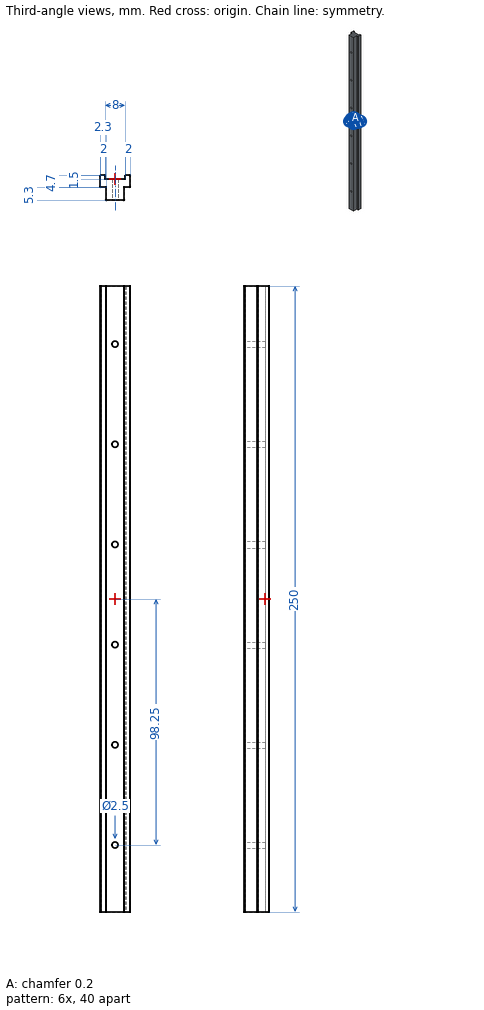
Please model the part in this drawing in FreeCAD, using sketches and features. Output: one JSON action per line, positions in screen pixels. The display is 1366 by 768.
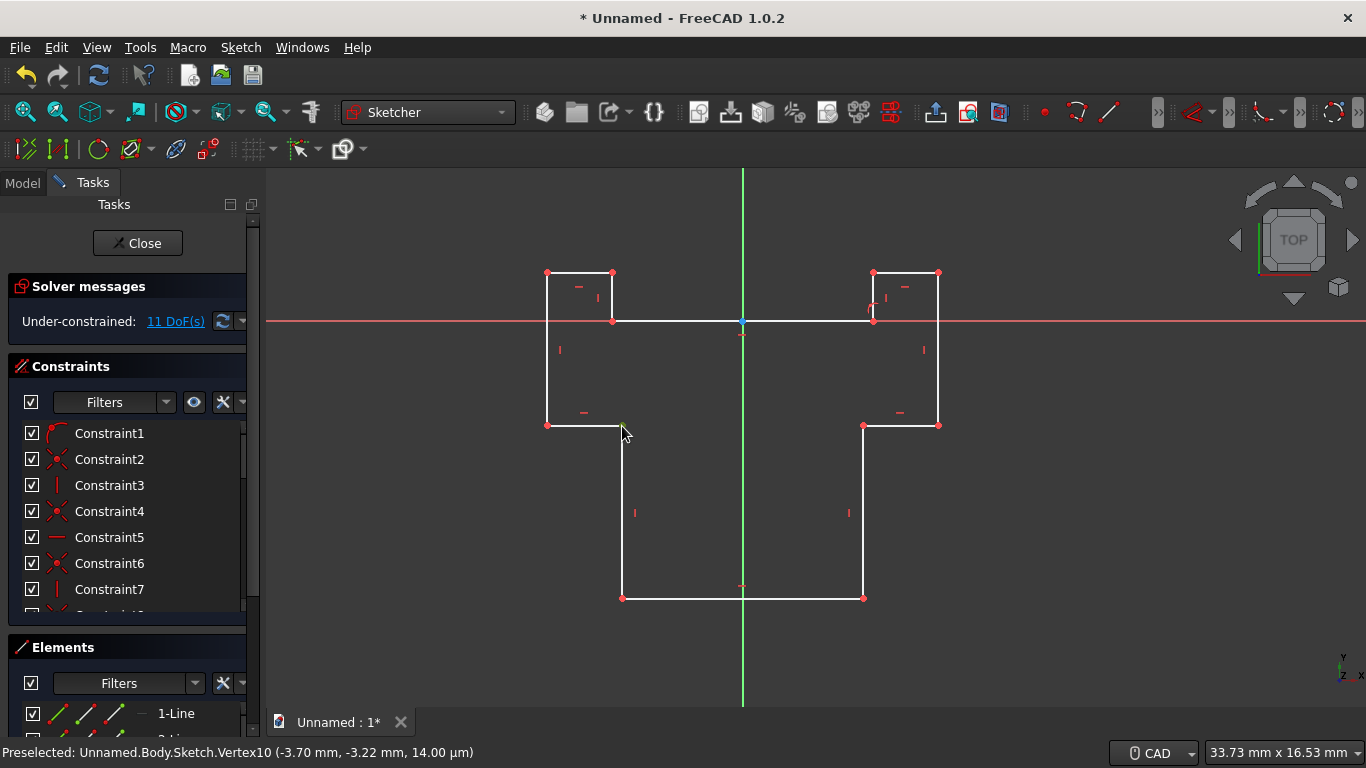
{"action": "left_click", "coordinate": [863, 426]}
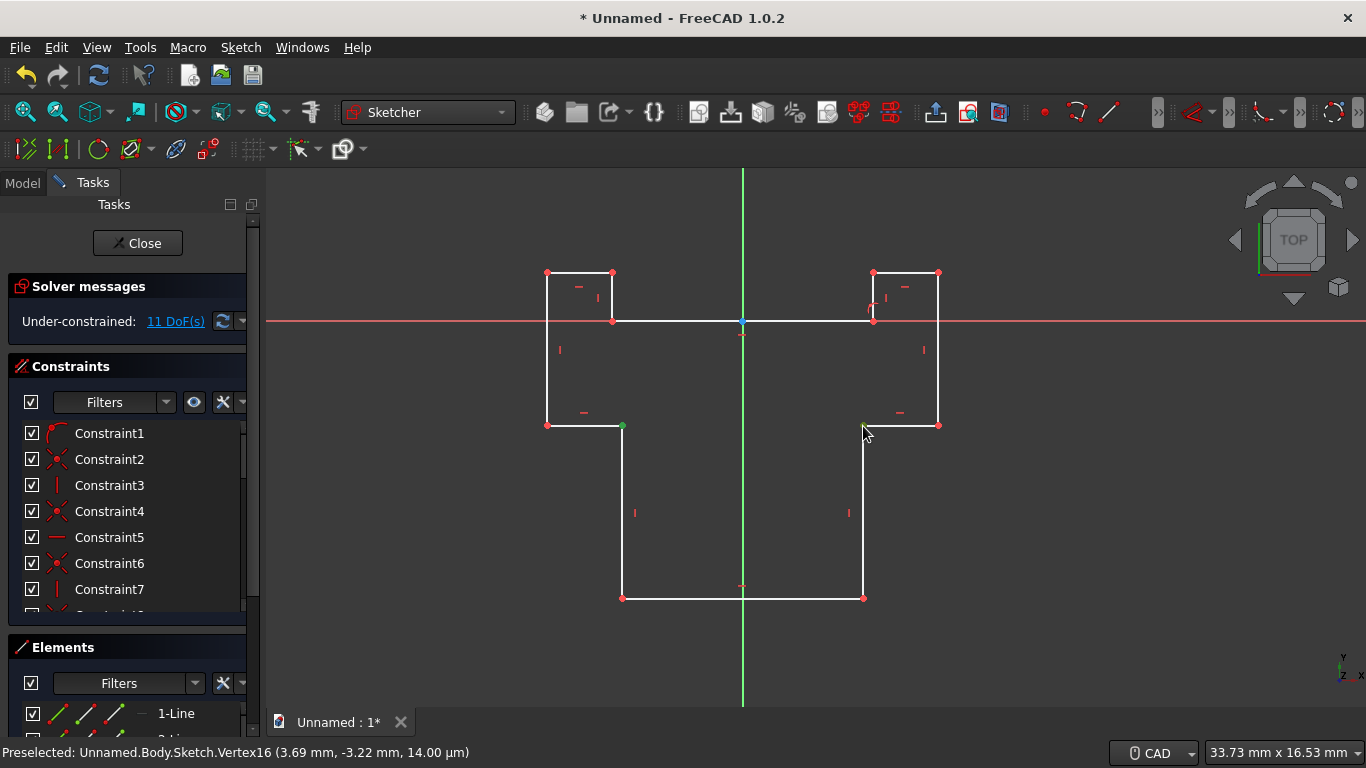
{"action": "left_click", "coordinate": [743, 644]}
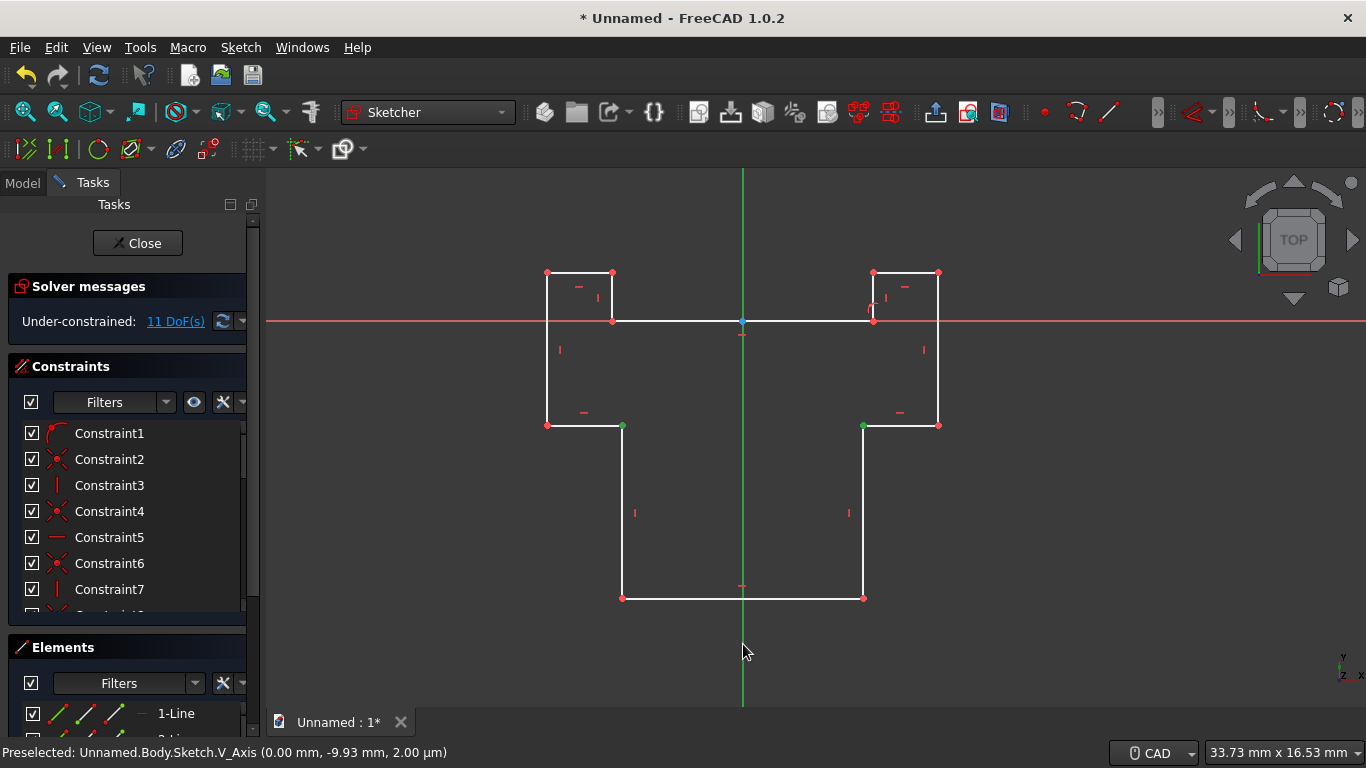
{"action": "key", "text": "s"}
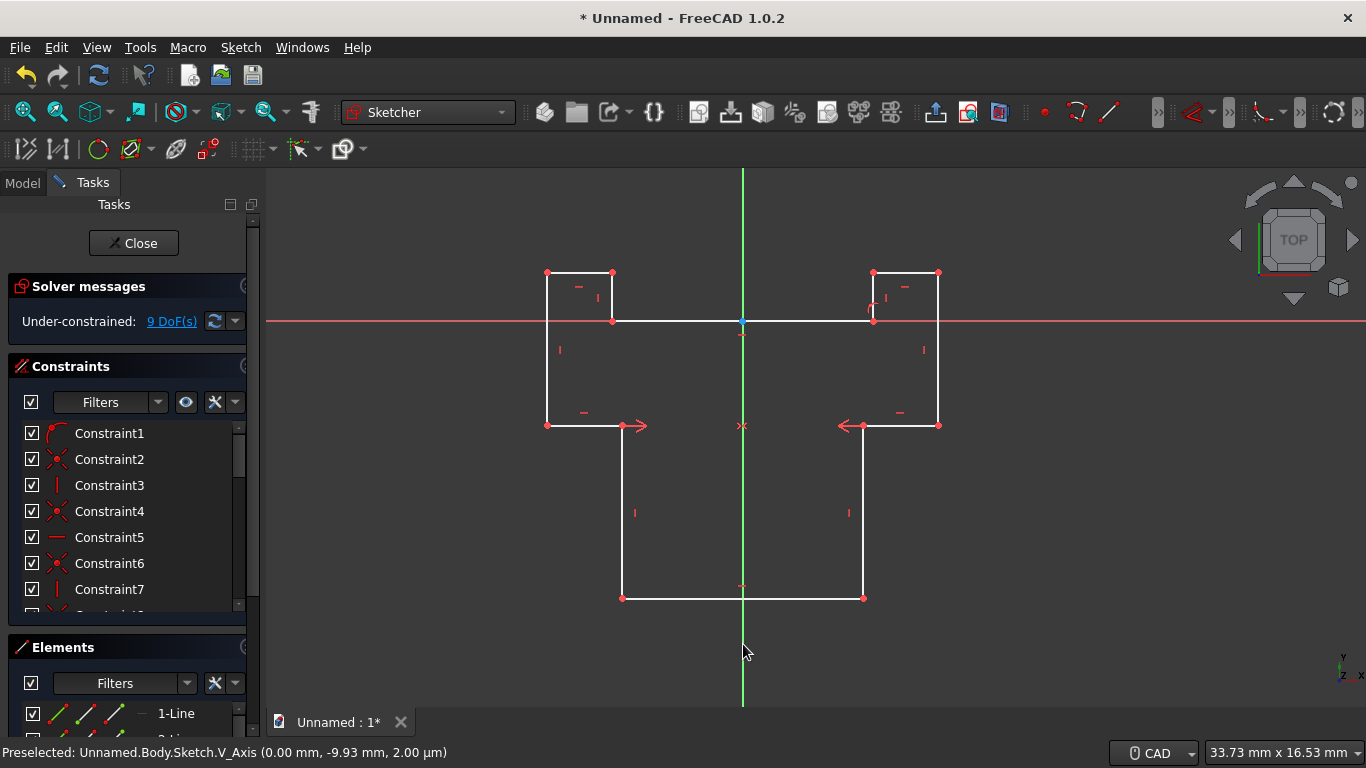
{"action": "left_click", "coordinate": [547, 273]}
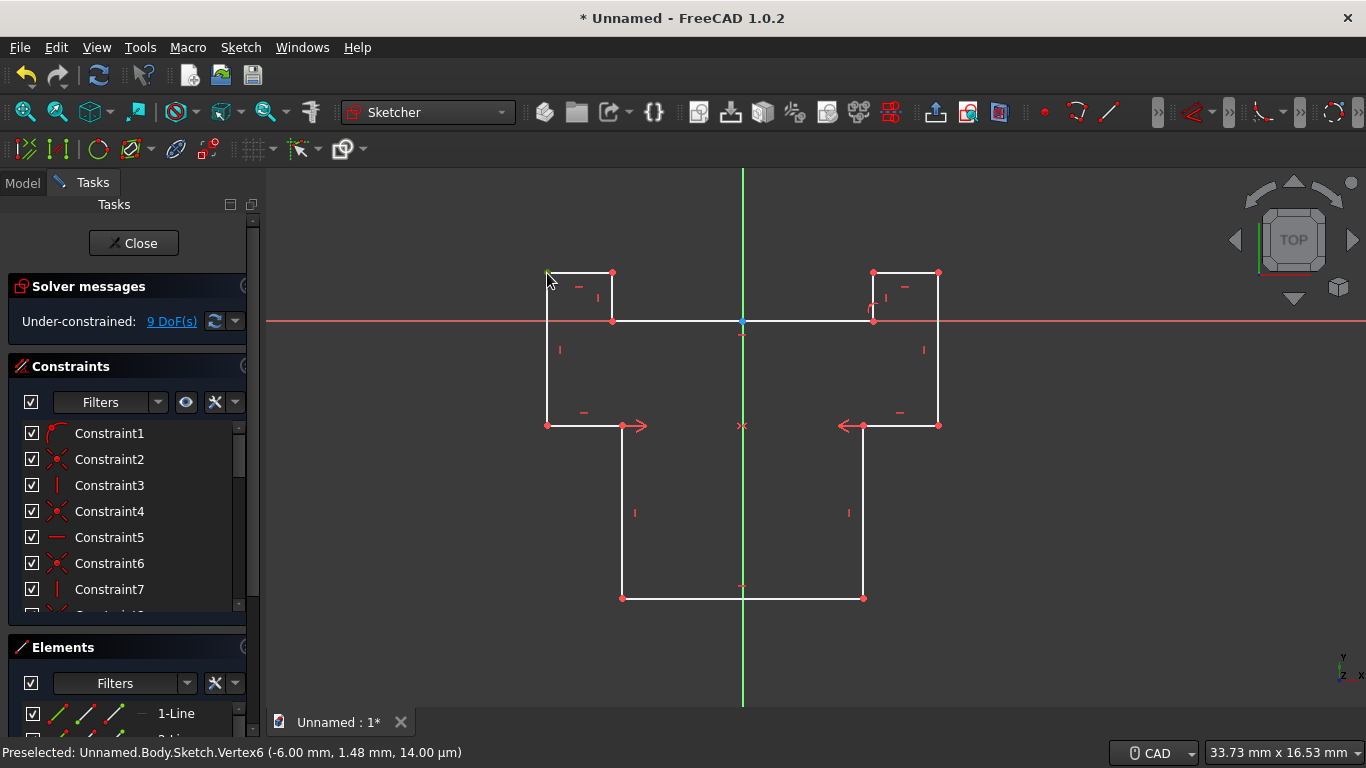
{"action": "left_click", "coordinate": [938, 273]}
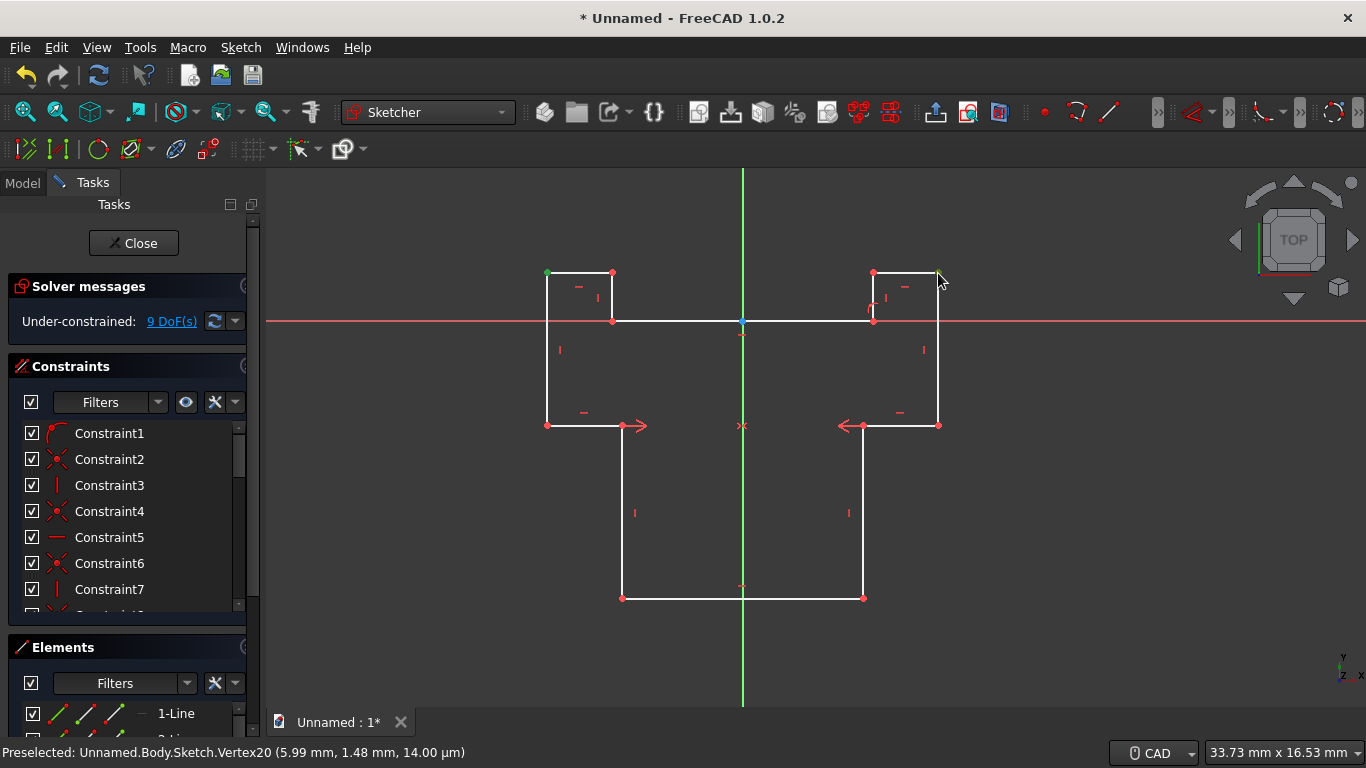
{"action": "left_click", "coordinate": [743, 644]}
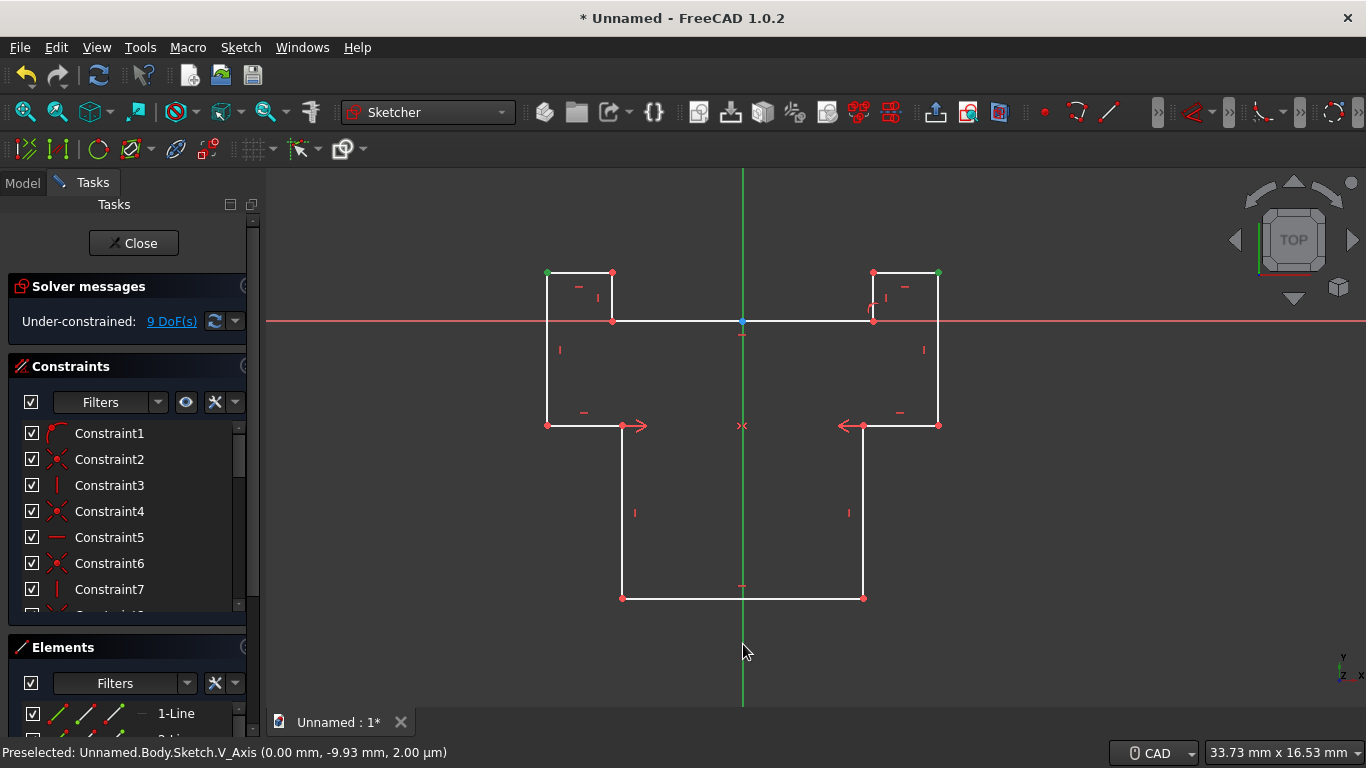
{"action": "key", "text": "s"}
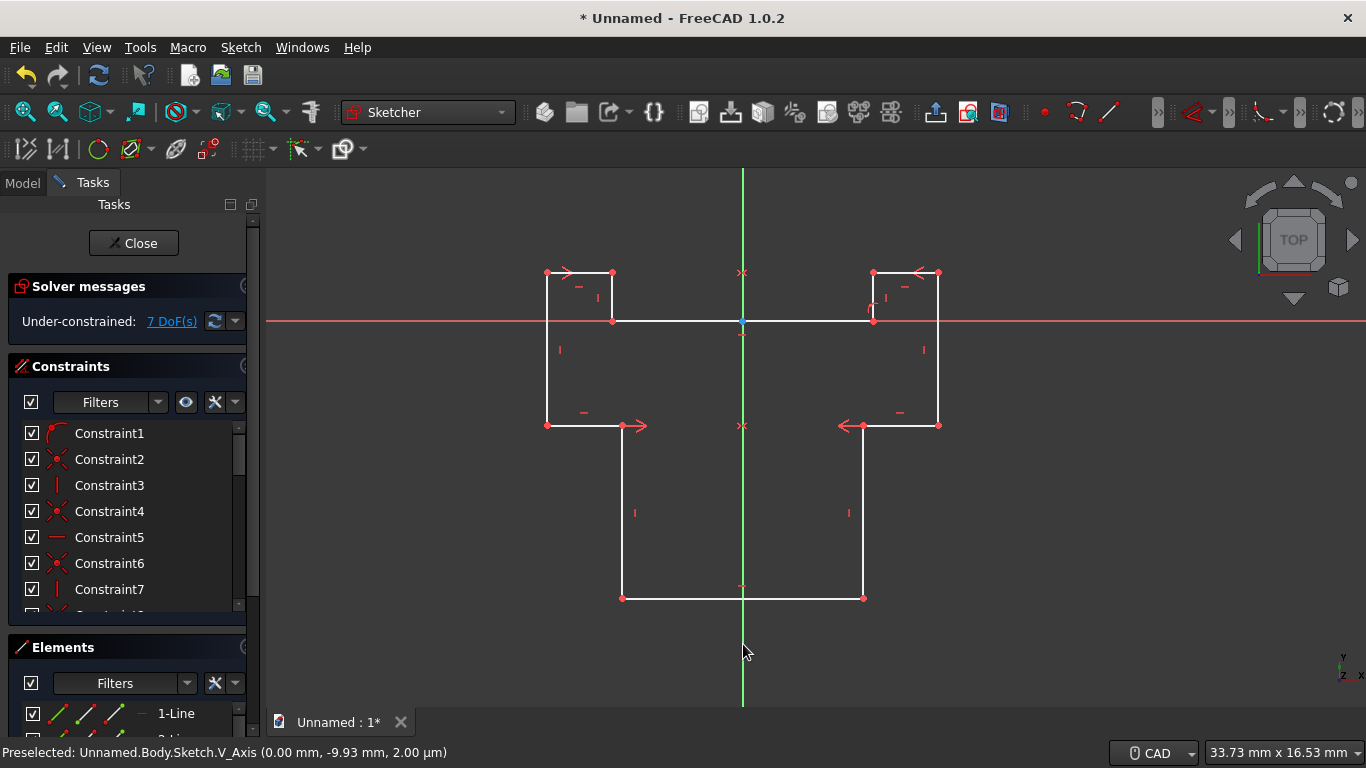
{"action": "left_click", "coordinate": [1192, 112]}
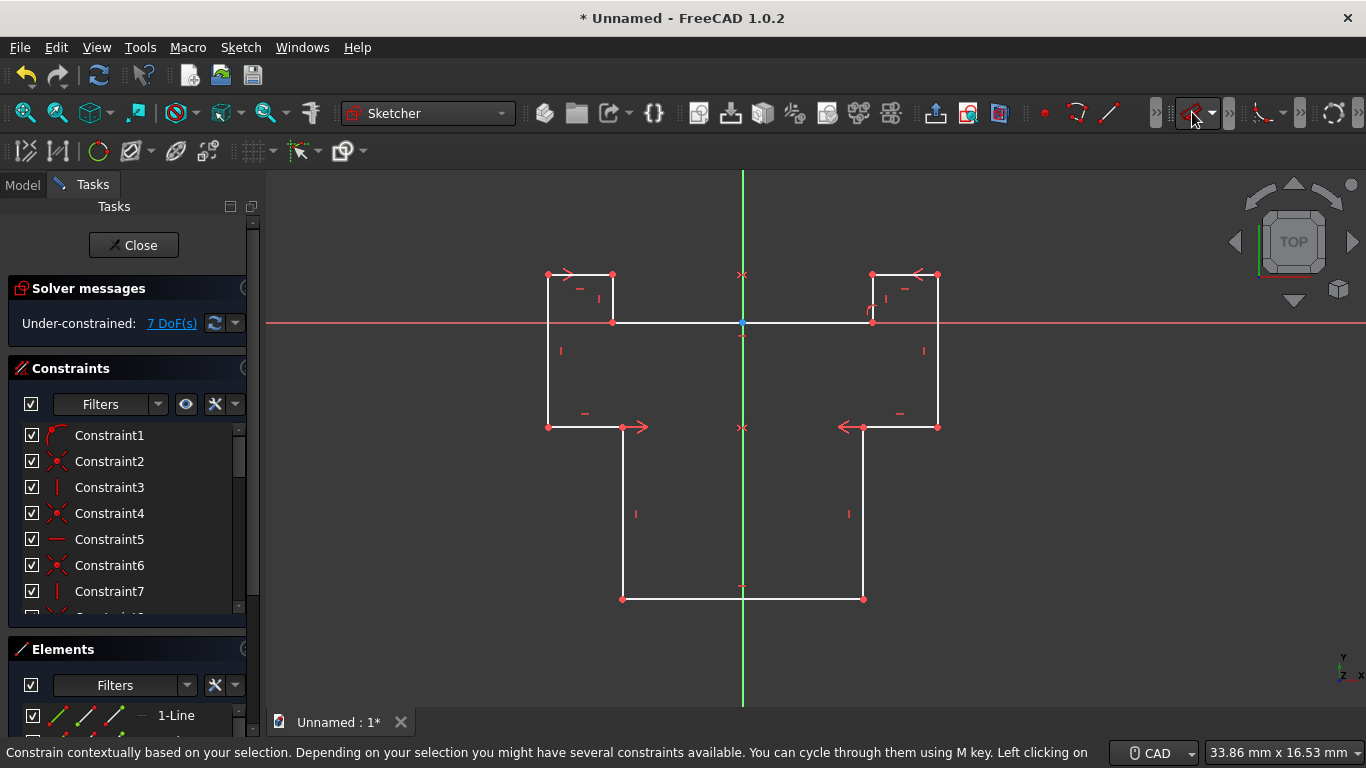
{"action": "left_click", "coordinate": [795, 323]}
{"action": "left_click", "coordinate": [683, 289]}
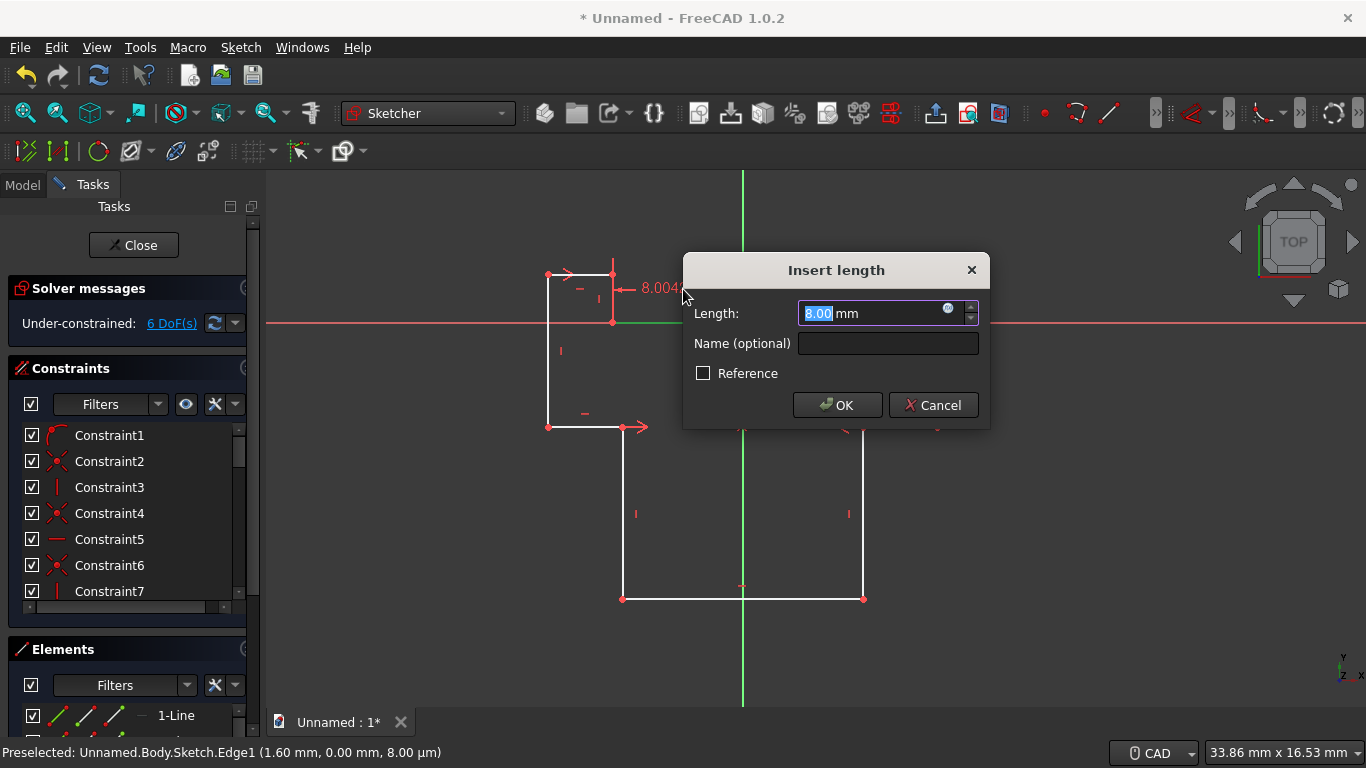
{"action": "type", "text": "8"}
{"action": "key", "text": "Return"}